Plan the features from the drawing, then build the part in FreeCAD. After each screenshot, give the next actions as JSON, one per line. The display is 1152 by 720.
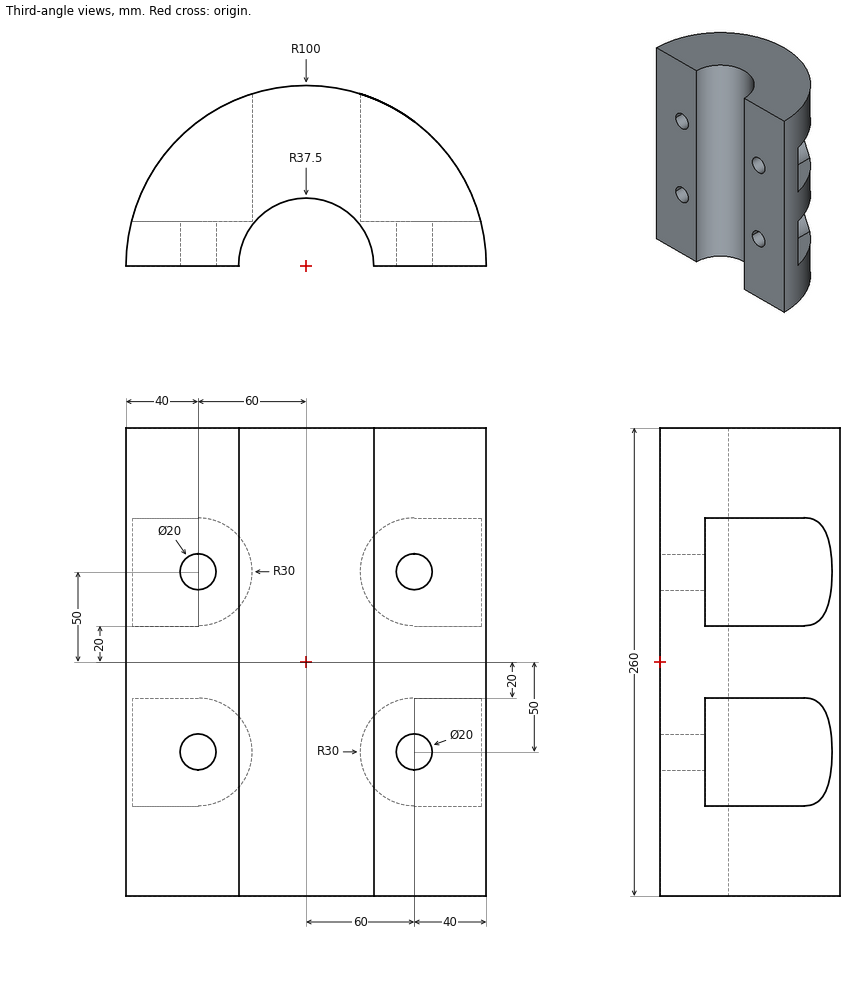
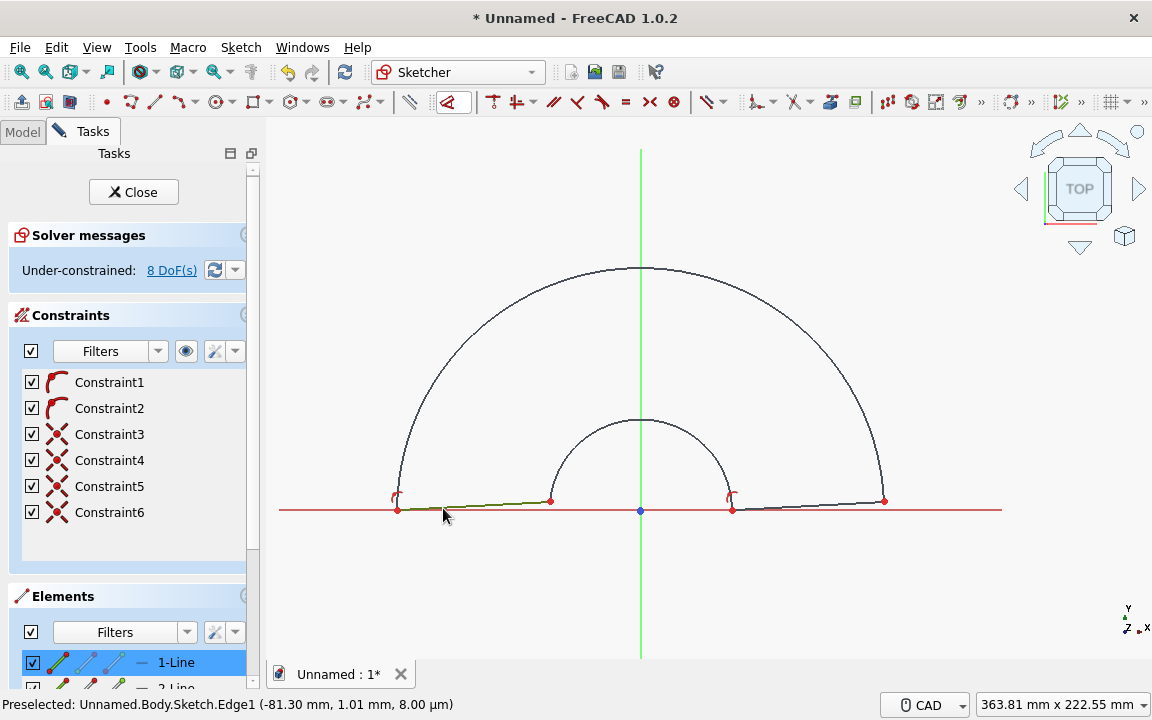
{"action": "key", "text": "h"}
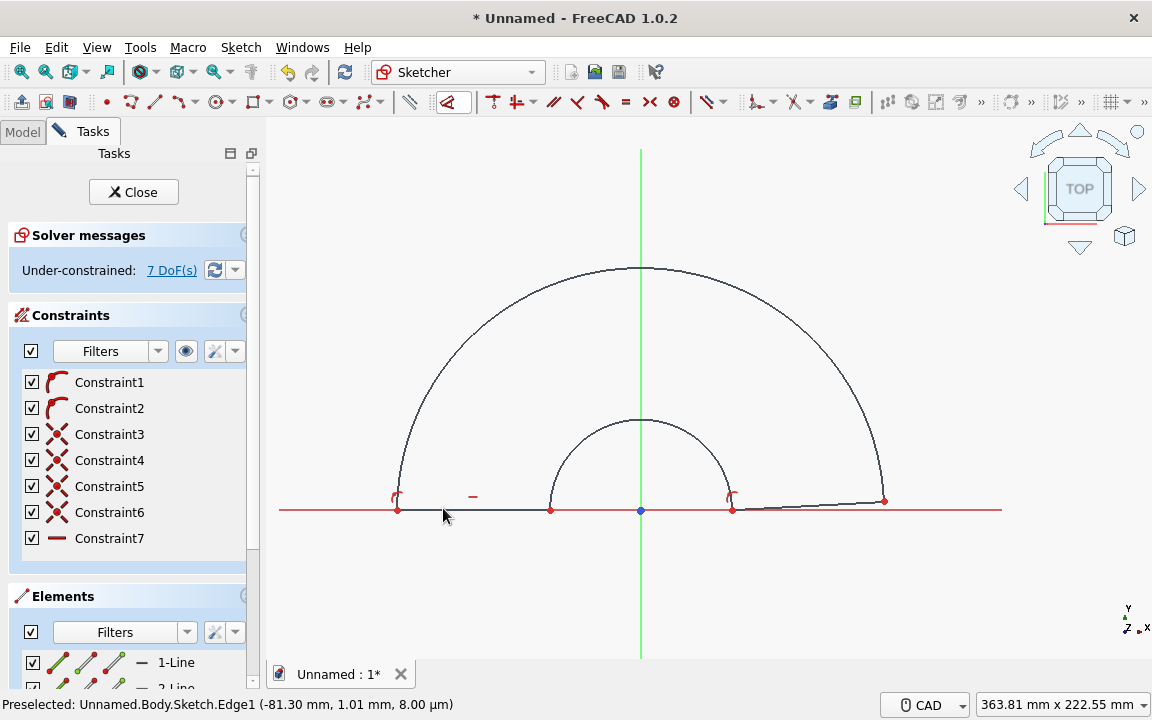
{"action": "left_click", "coordinate": [778, 508]}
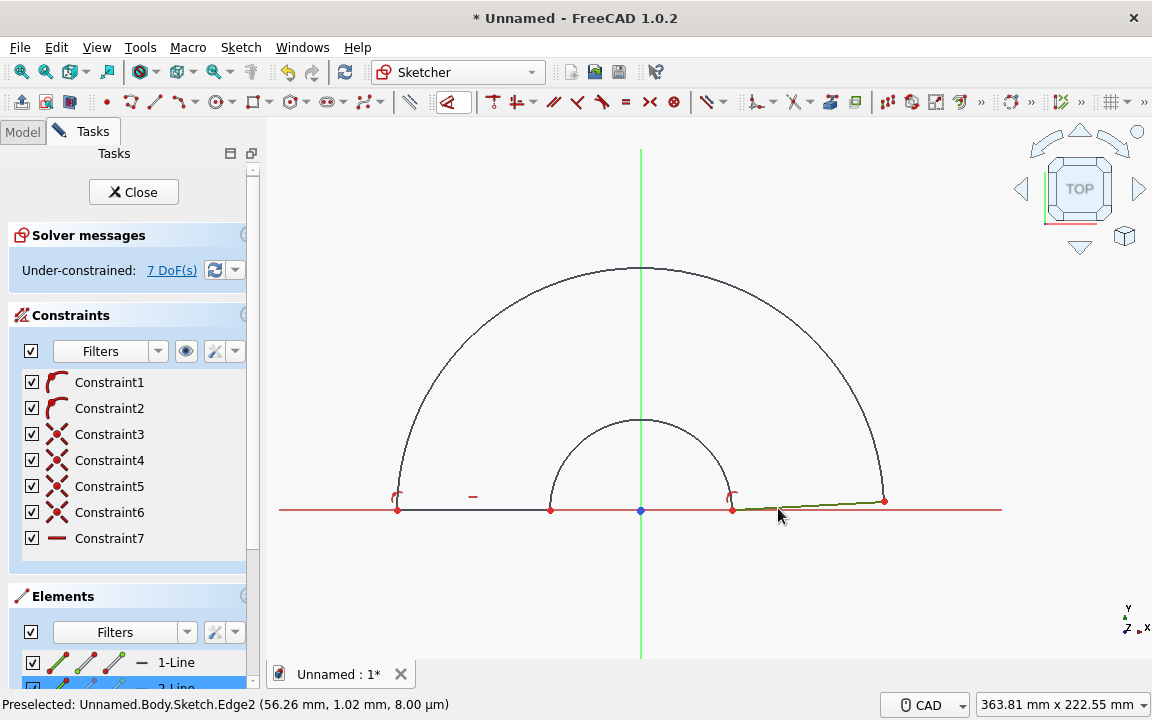
{"action": "left_click", "coordinate": [536, 102]}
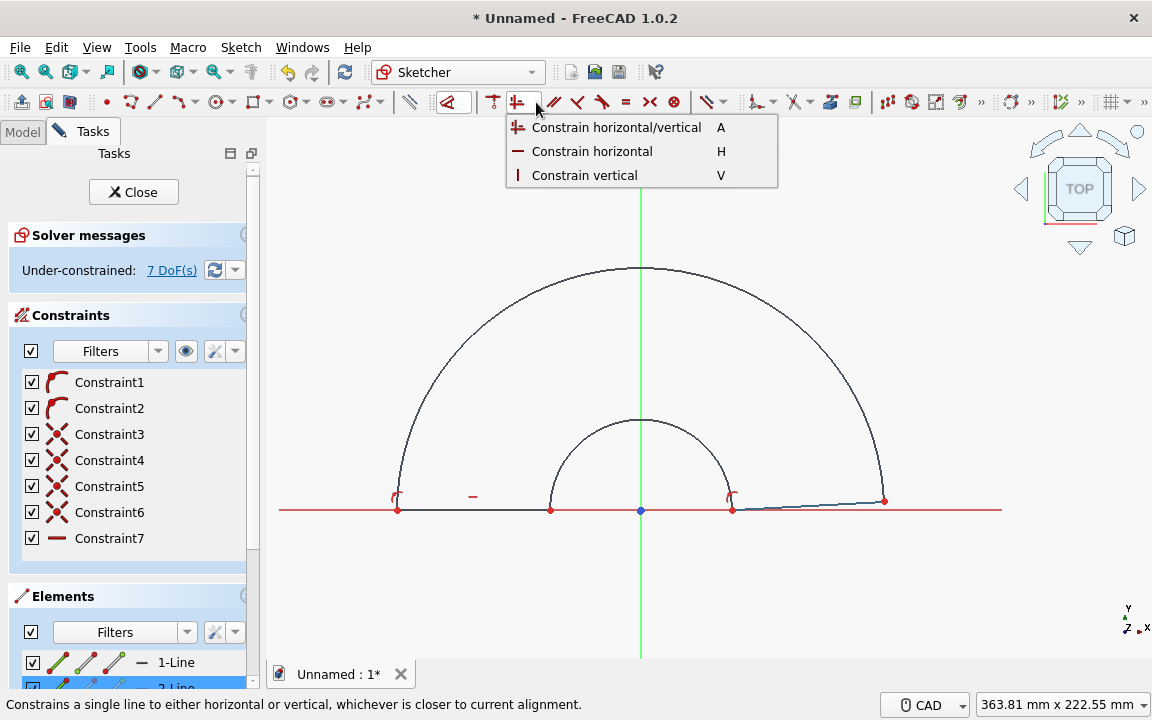
{"action": "left_click", "coordinate": [642, 151]}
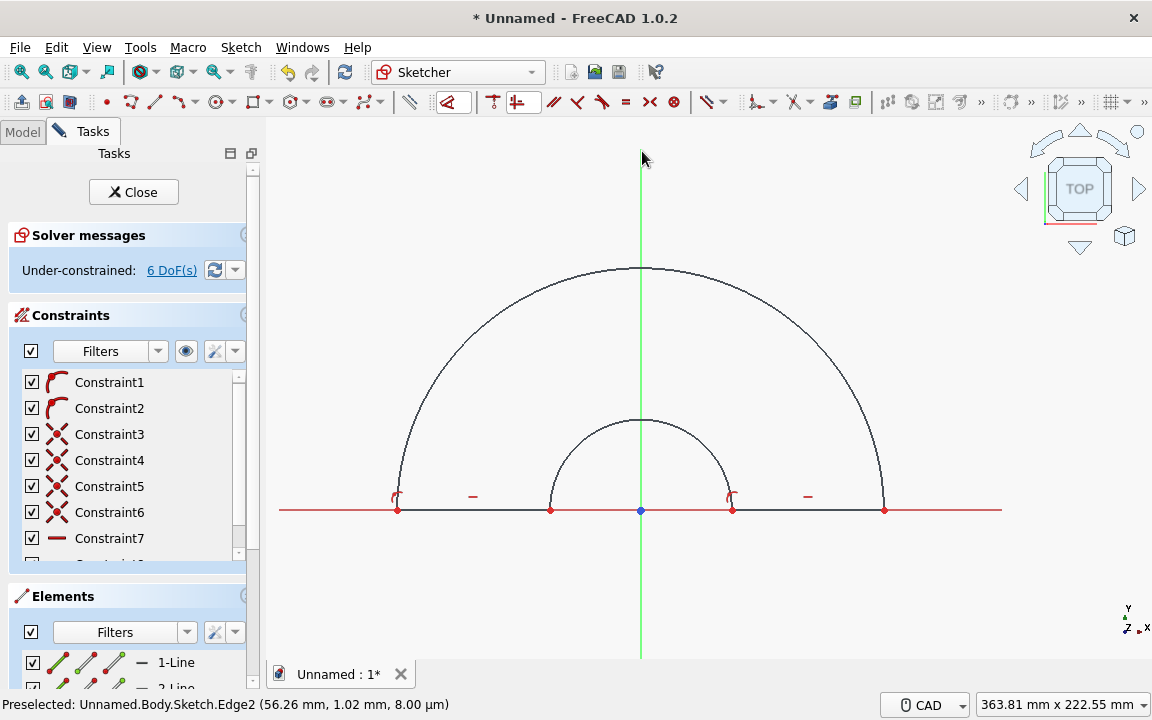
{"action": "left_click", "coordinate": [694, 437]}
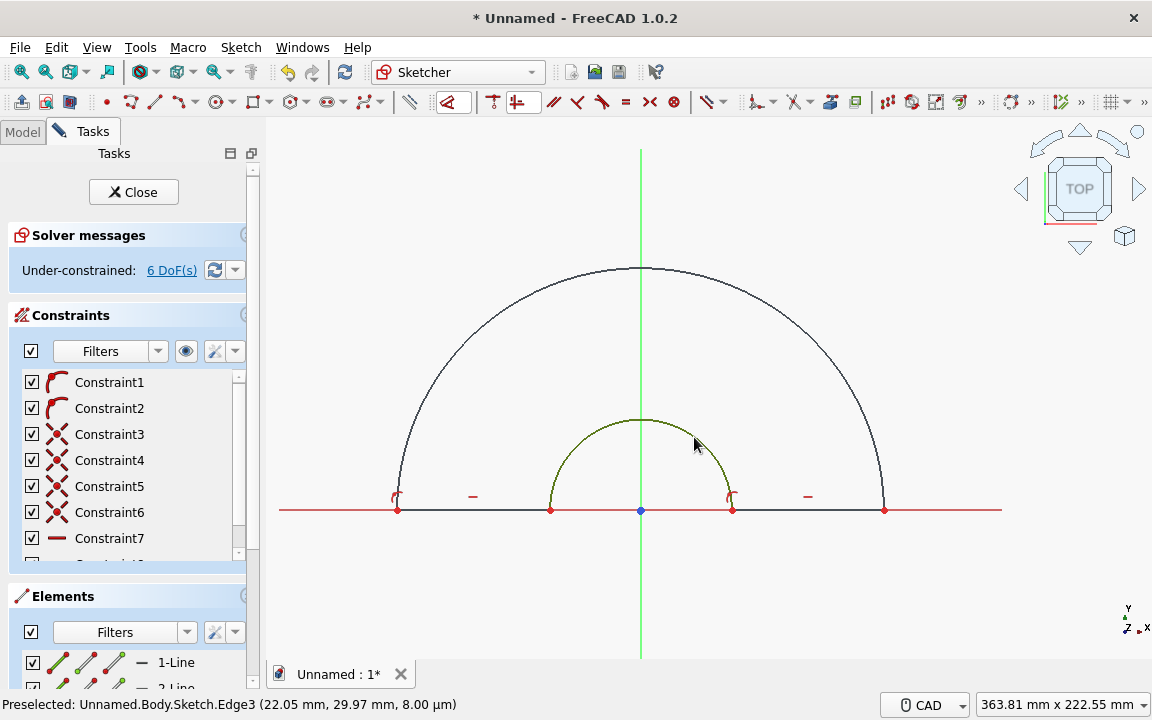
{"action": "left_click", "coordinate": [783, 314]}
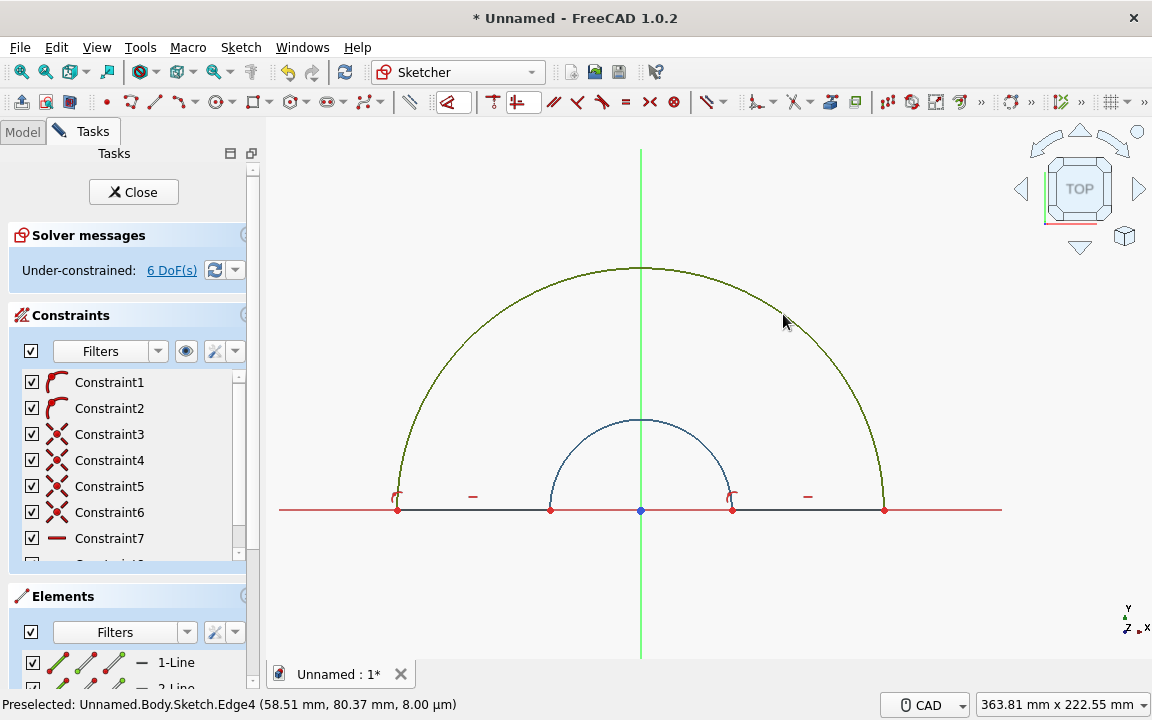
{"action": "key", "text": "c"}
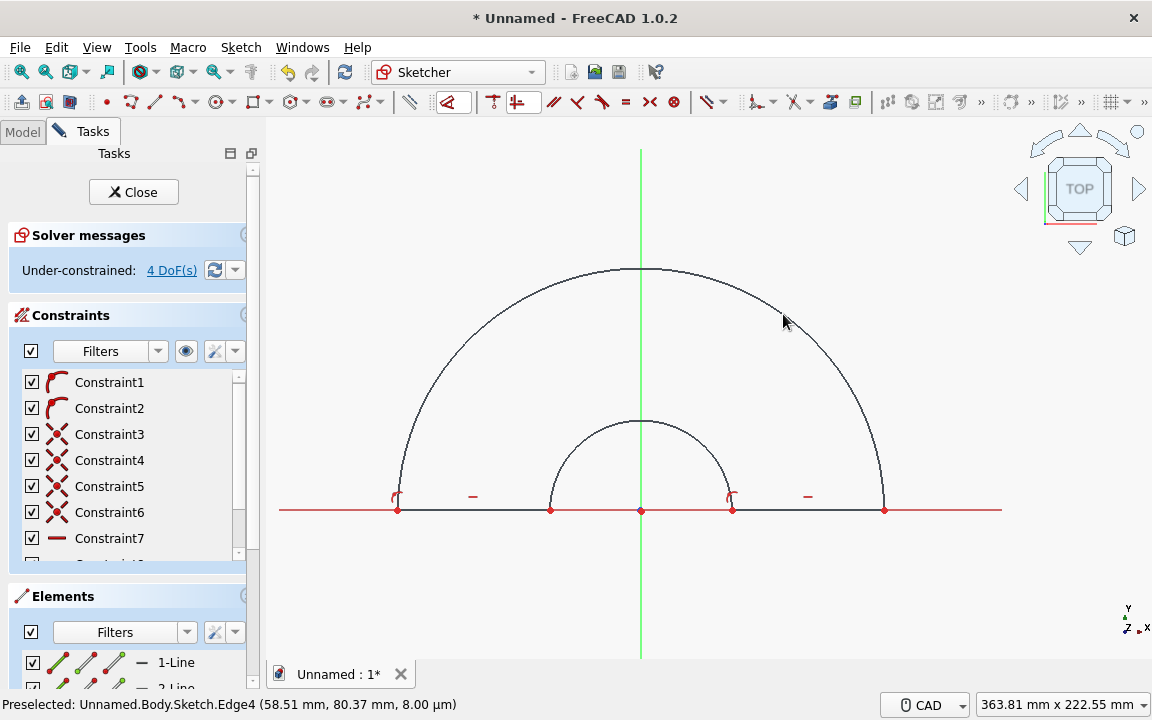
{"action": "left_click_drag", "start_coordinate": [631, 500], "coordinate": [651, 522]}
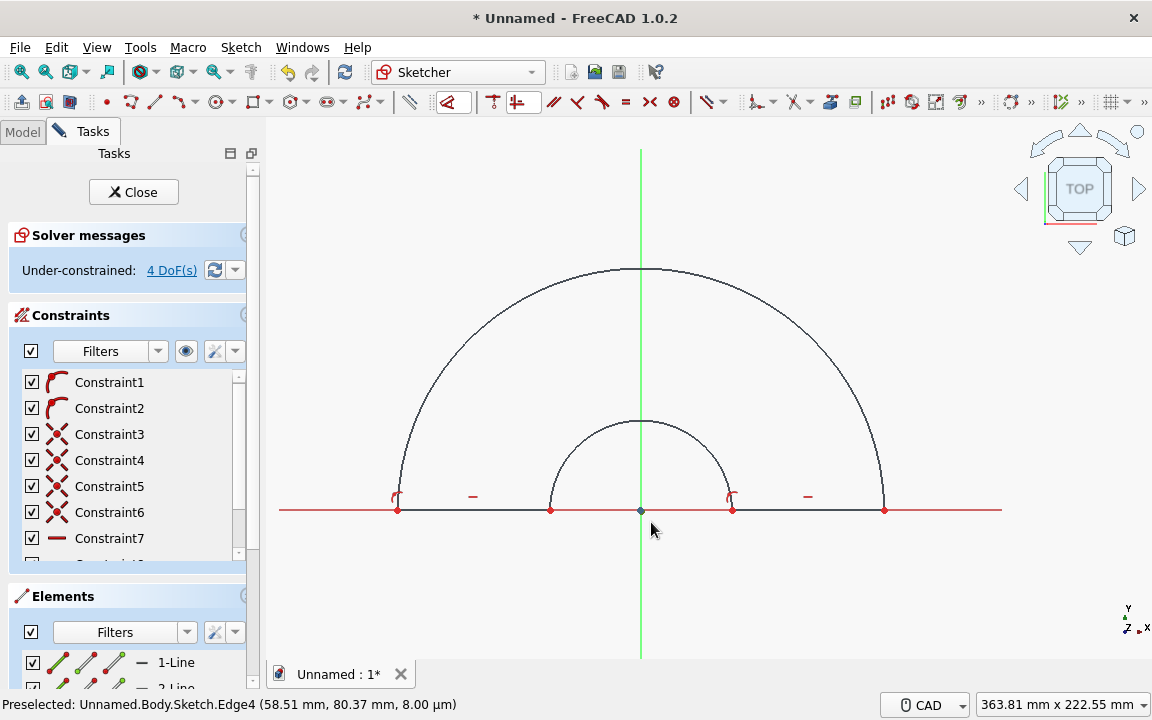
{"action": "key", "text": "c"}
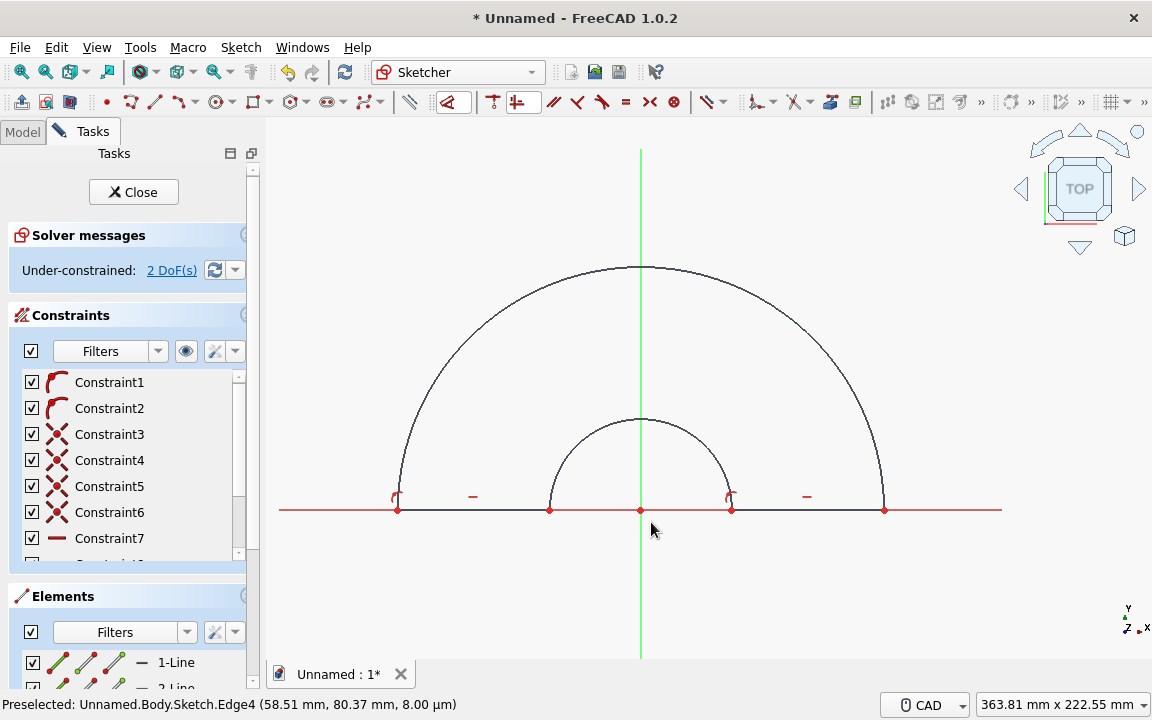
{"action": "left_click", "coordinate": [694, 437]}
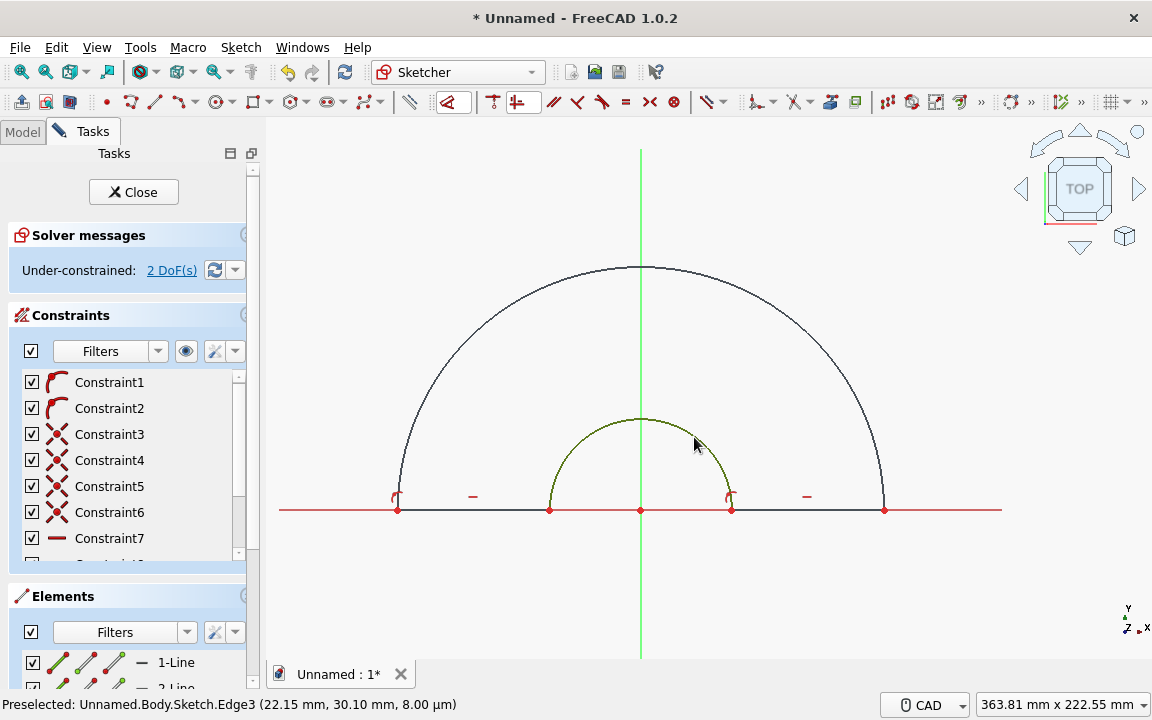
{"action": "key", "text": "k r"}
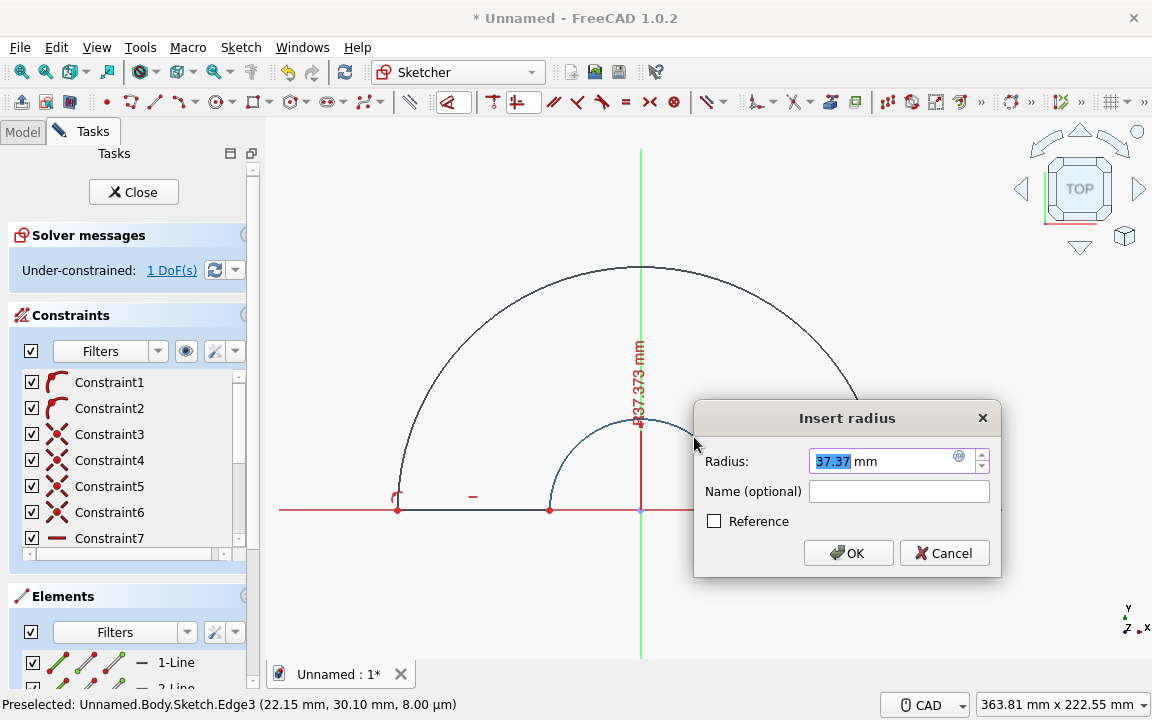
{"action": "type", "text": "37.5"}
{"action": "key", "text": "Return"}